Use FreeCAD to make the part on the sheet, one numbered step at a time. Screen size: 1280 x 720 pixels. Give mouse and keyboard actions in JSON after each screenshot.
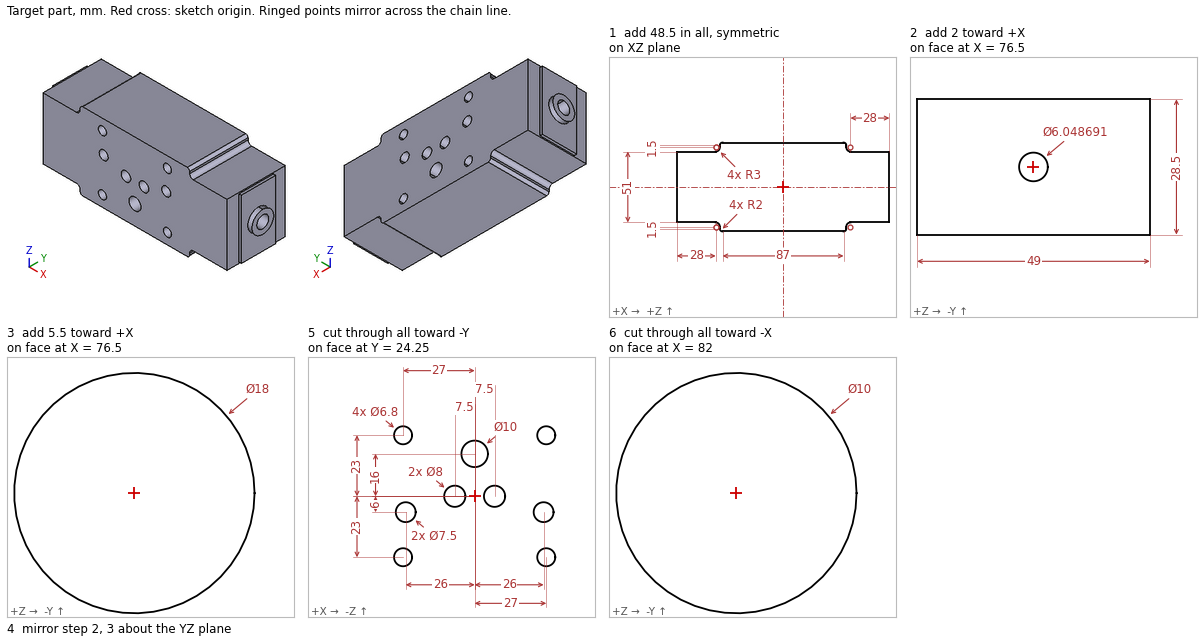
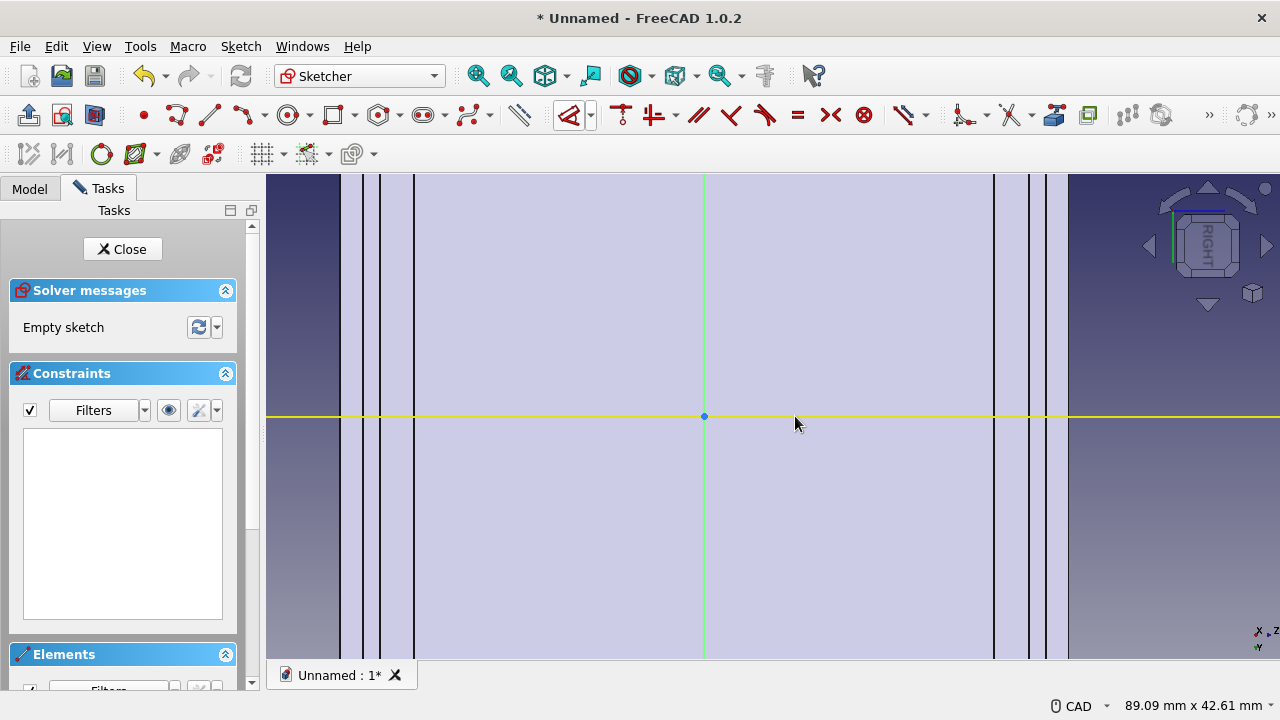
{"action": "left_click", "coordinate": [354, 116]}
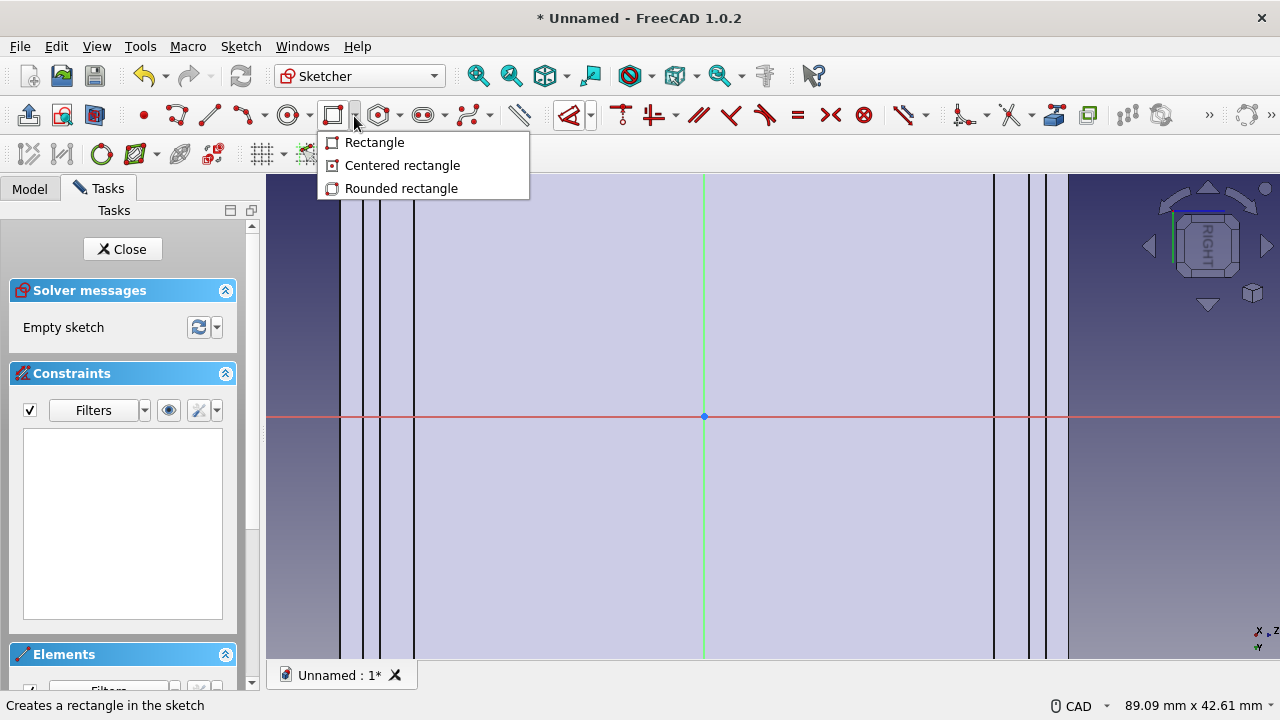
{"action": "left_click", "coordinate": [424, 166]}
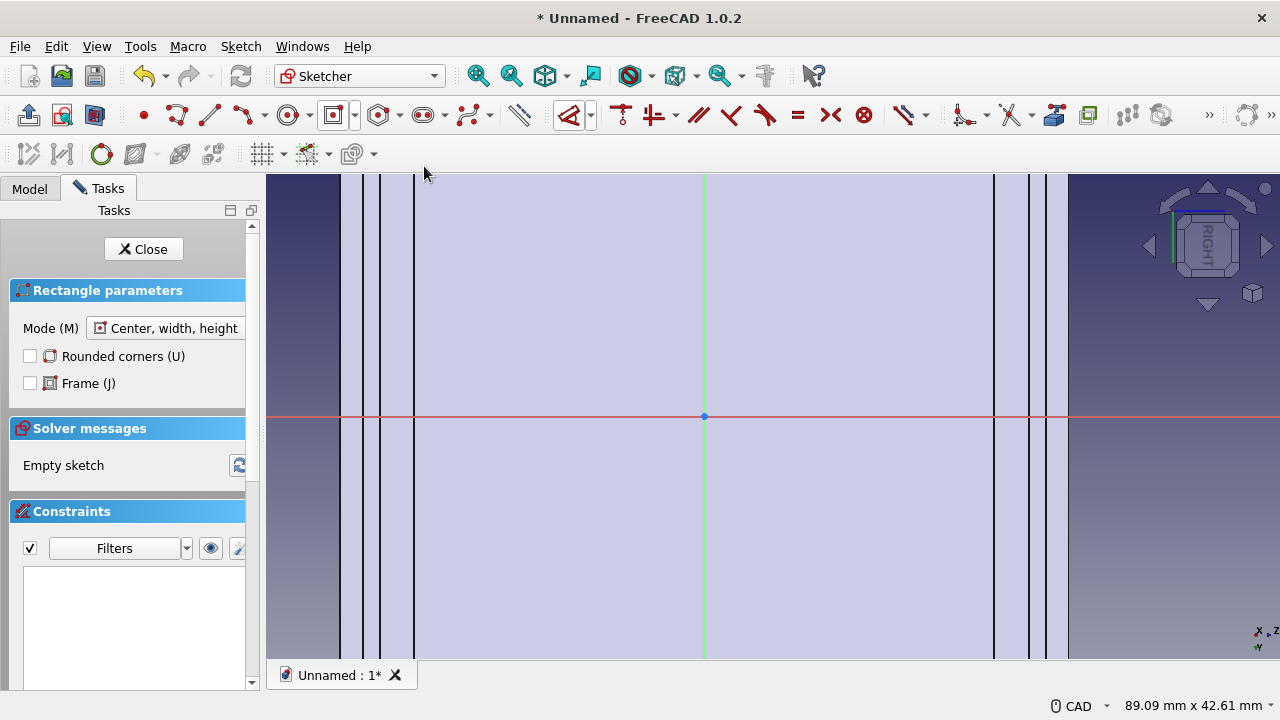
{"action": "left_click", "coordinate": [704, 416]}
{"action": "left_click", "coordinate": [983, 254]}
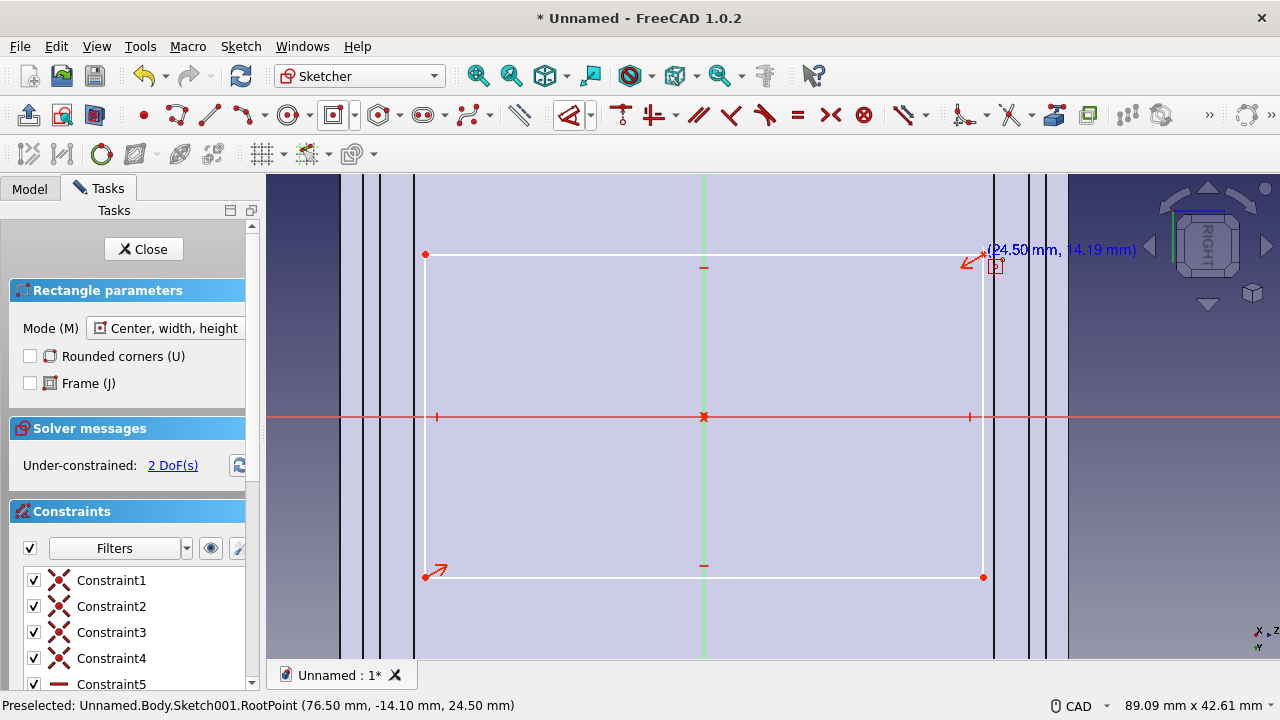
{"action": "left_click", "coordinate": [288, 116]}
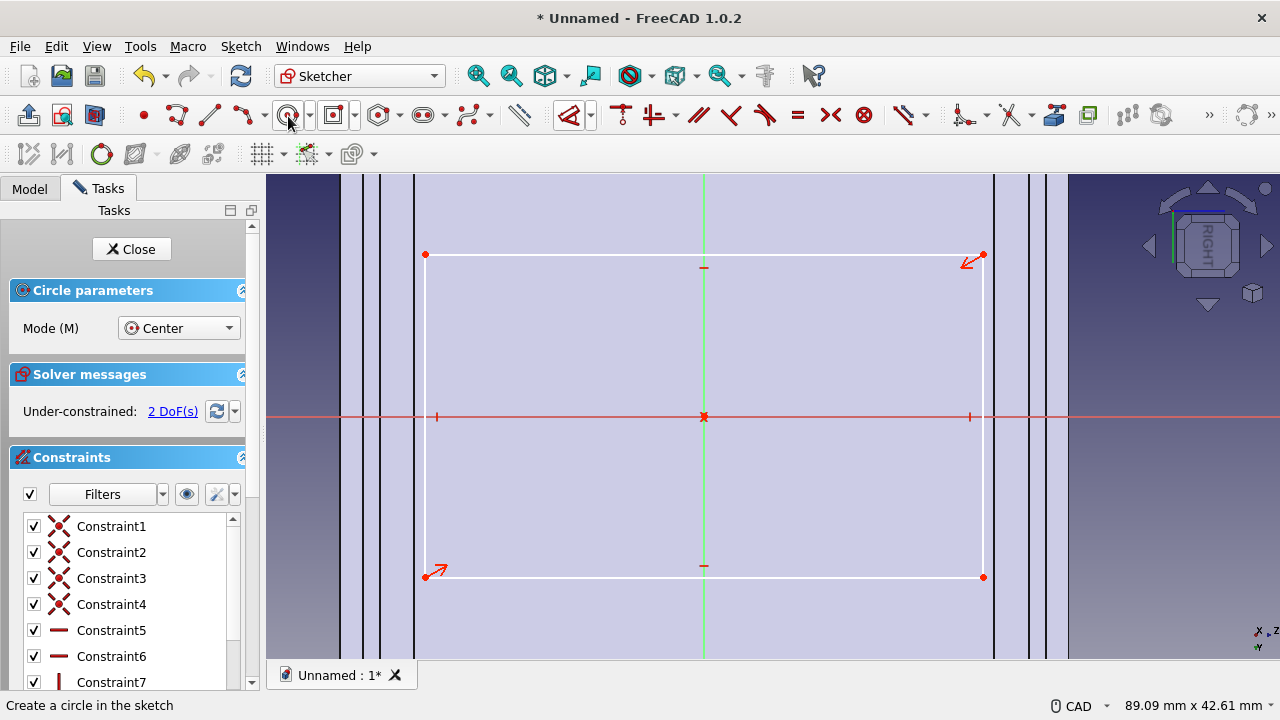
{"action": "left_click", "coordinate": [704, 416]}
{"action": "left_click", "coordinate": [729, 392]}
{"action": "key", "text": "Escape"}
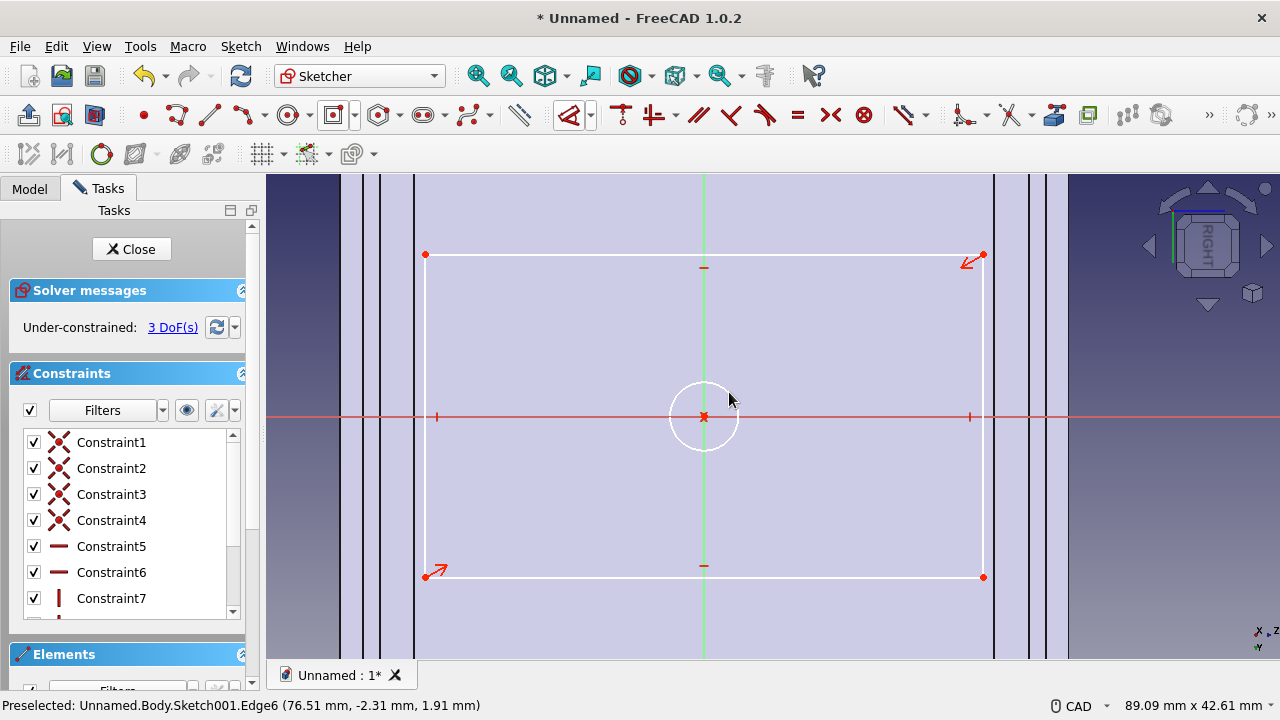
{"action": "left_click", "coordinate": [728, 392]}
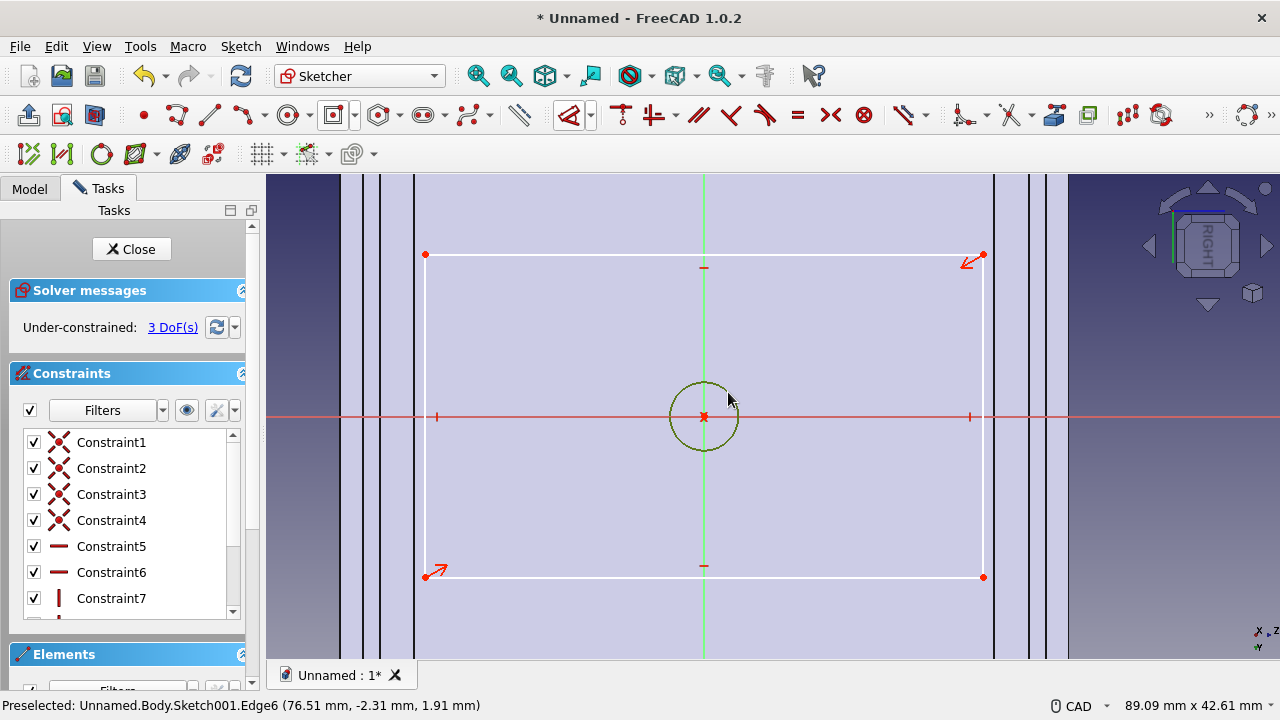
{"action": "left_click", "coordinate": [590, 116]}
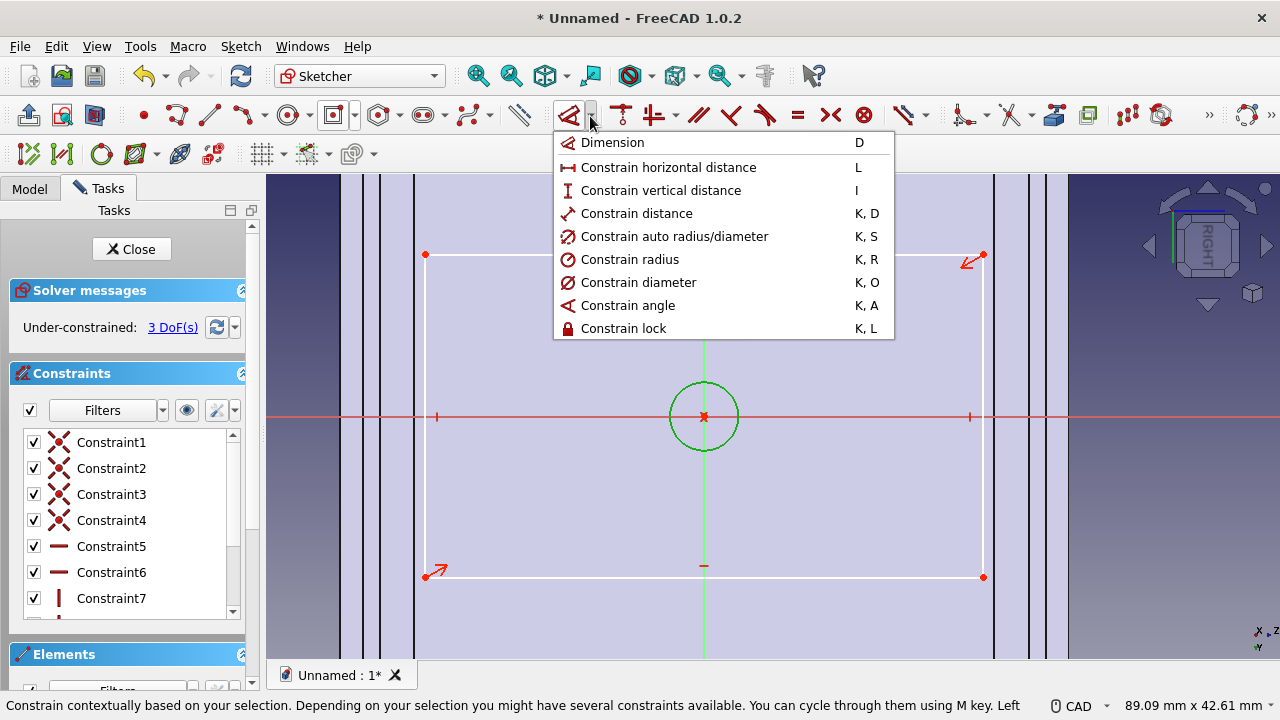
{"action": "left_click", "coordinate": [724, 282]}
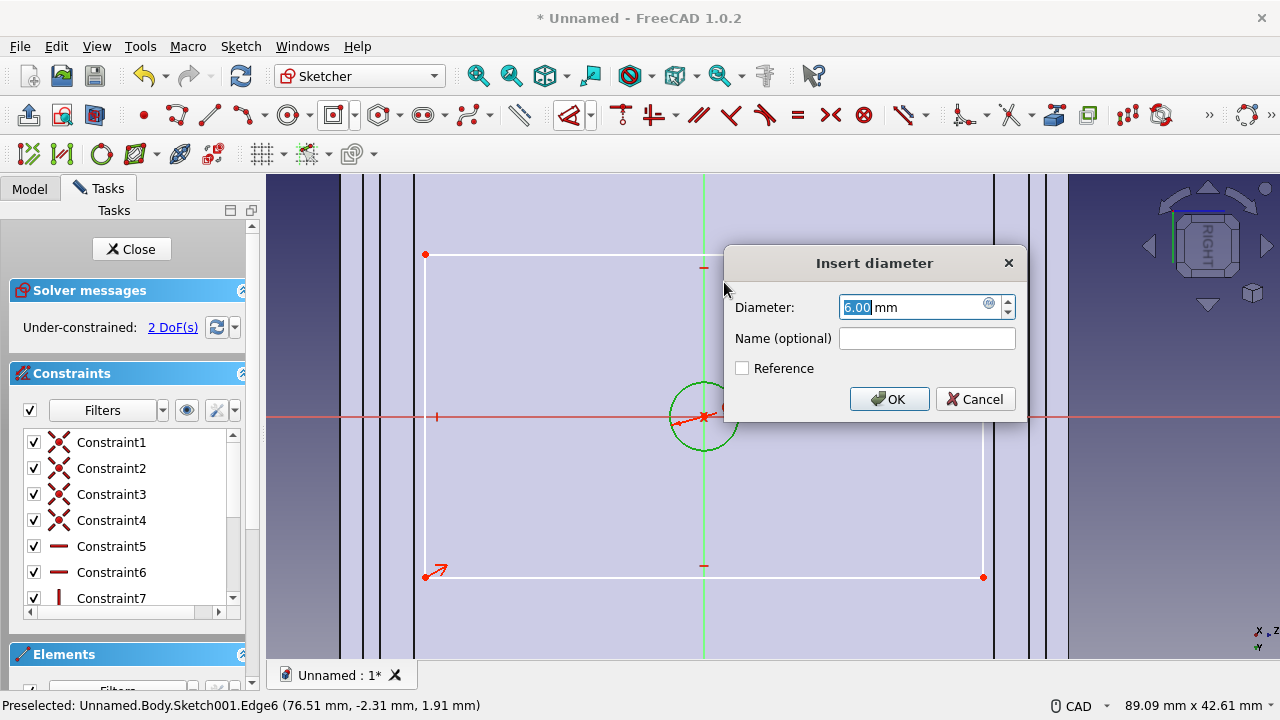
{"action": "type", "text": "6.048691"}
{"action": "key", "text": "Return"}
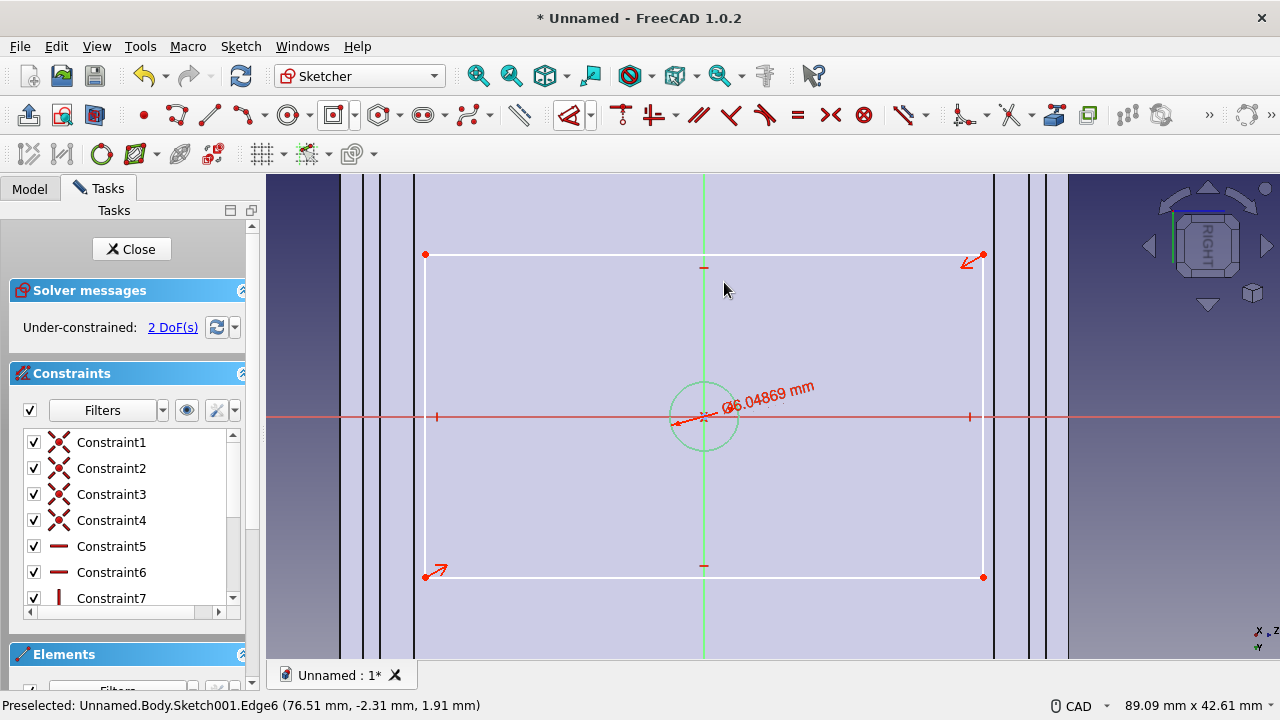
{"action": "left_click", "coordinate": [593, 578]}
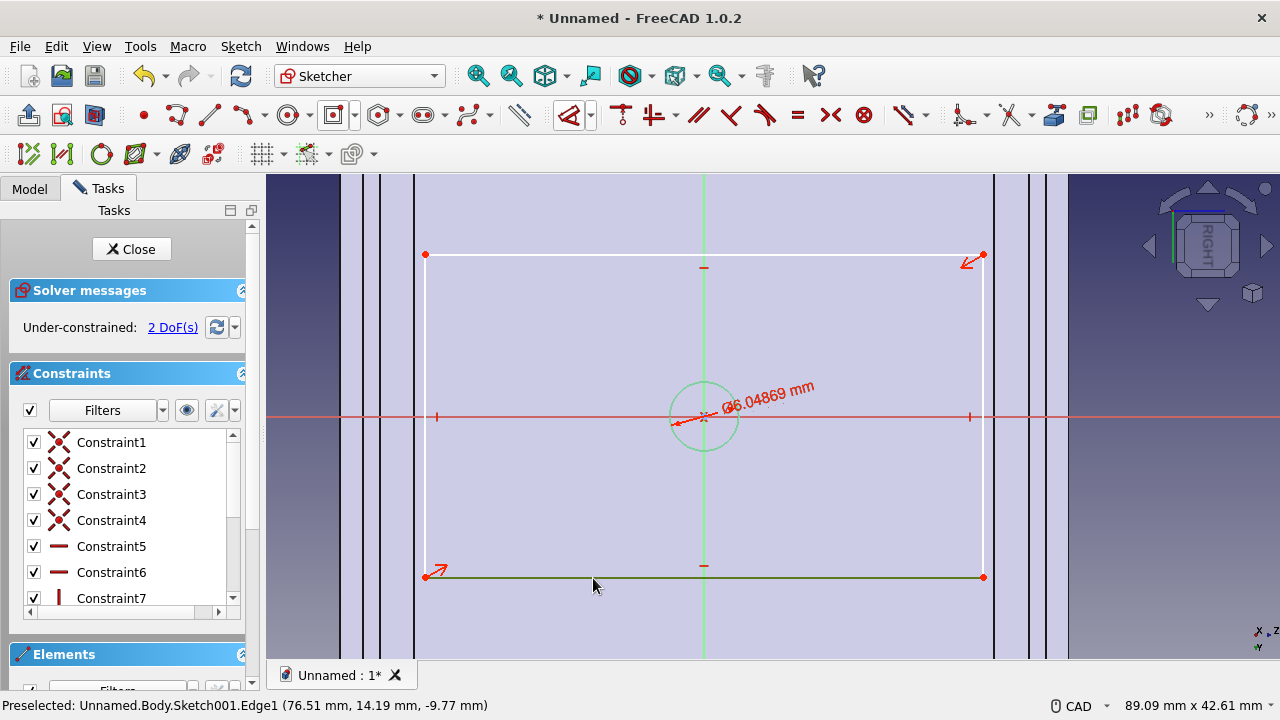
{"action": "left_click", "coordinate": [590, 116]}